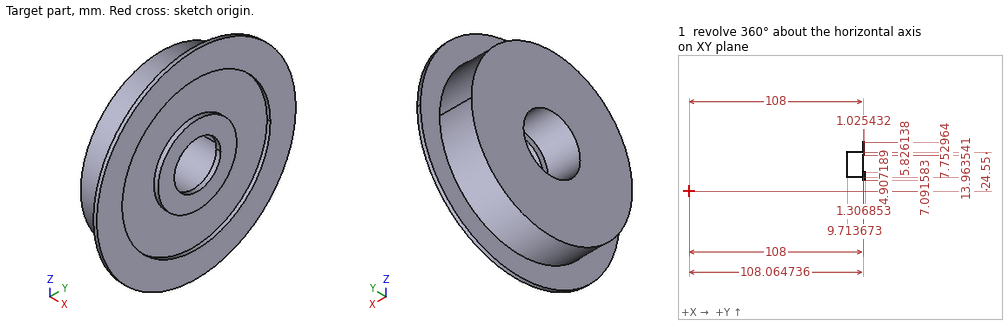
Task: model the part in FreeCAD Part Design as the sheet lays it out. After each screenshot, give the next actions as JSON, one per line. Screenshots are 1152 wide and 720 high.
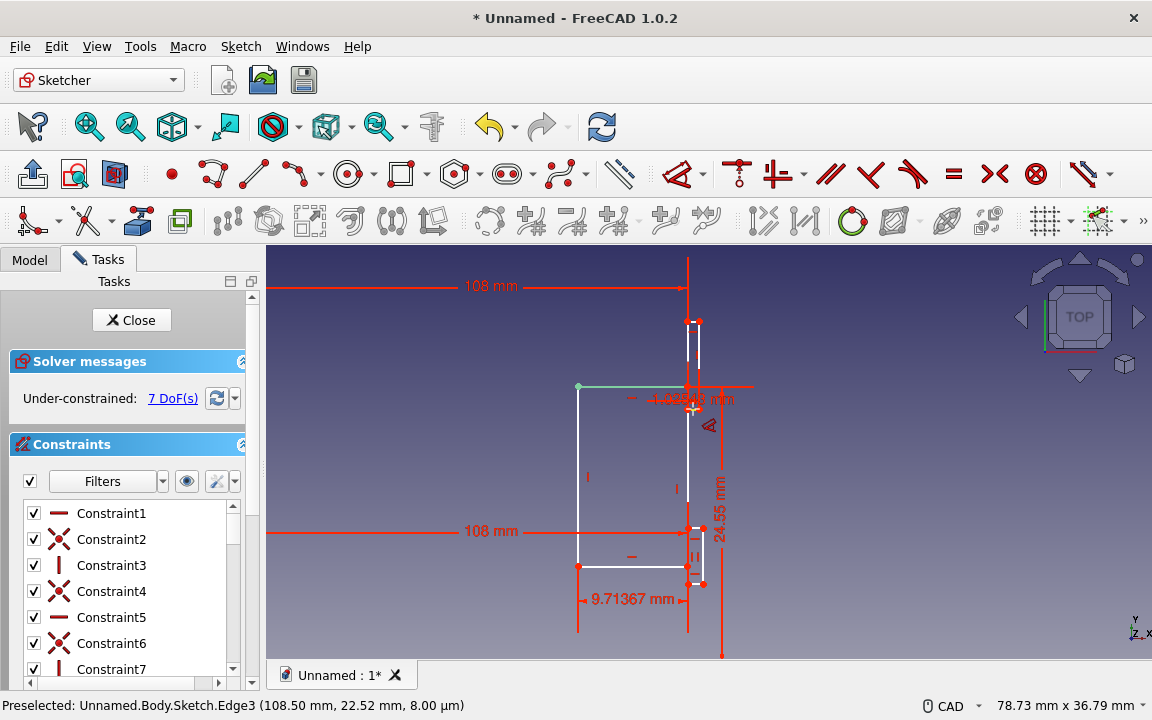
{"action": "left_click", "coordinate": [699, 383]}
{"action": "left_click", "coordinate": [733, 366]}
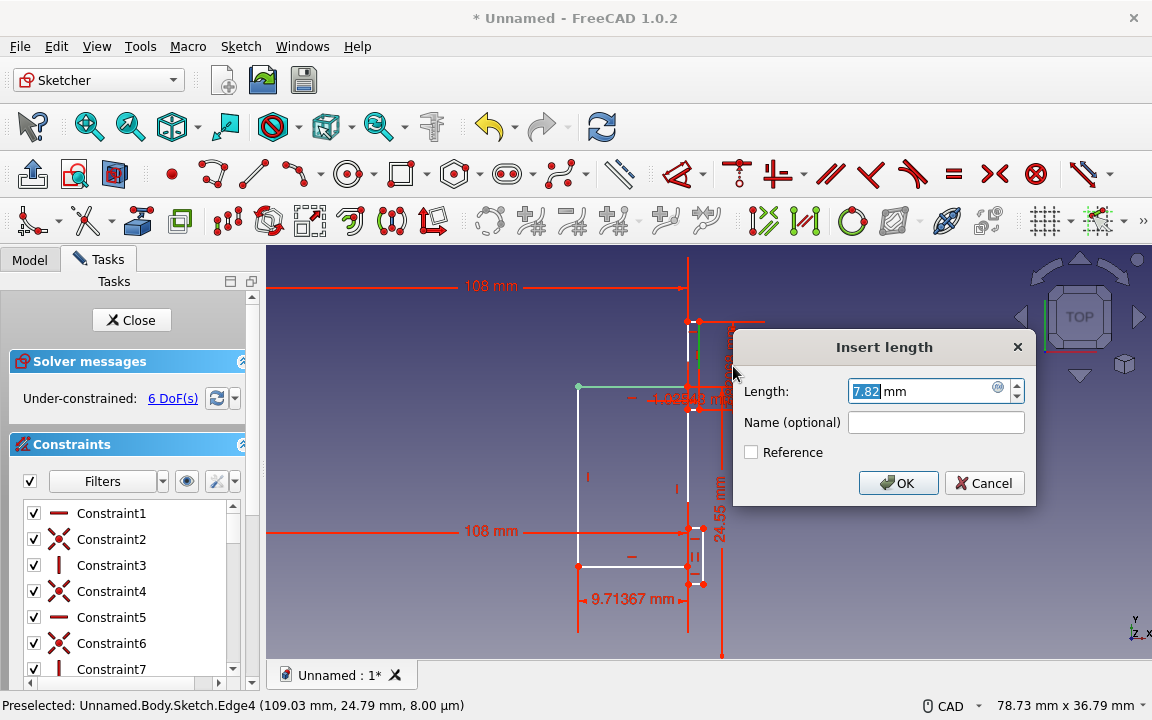
{"action": "type", "text": "7.752964"}
{"action": "key", "text": "Return"}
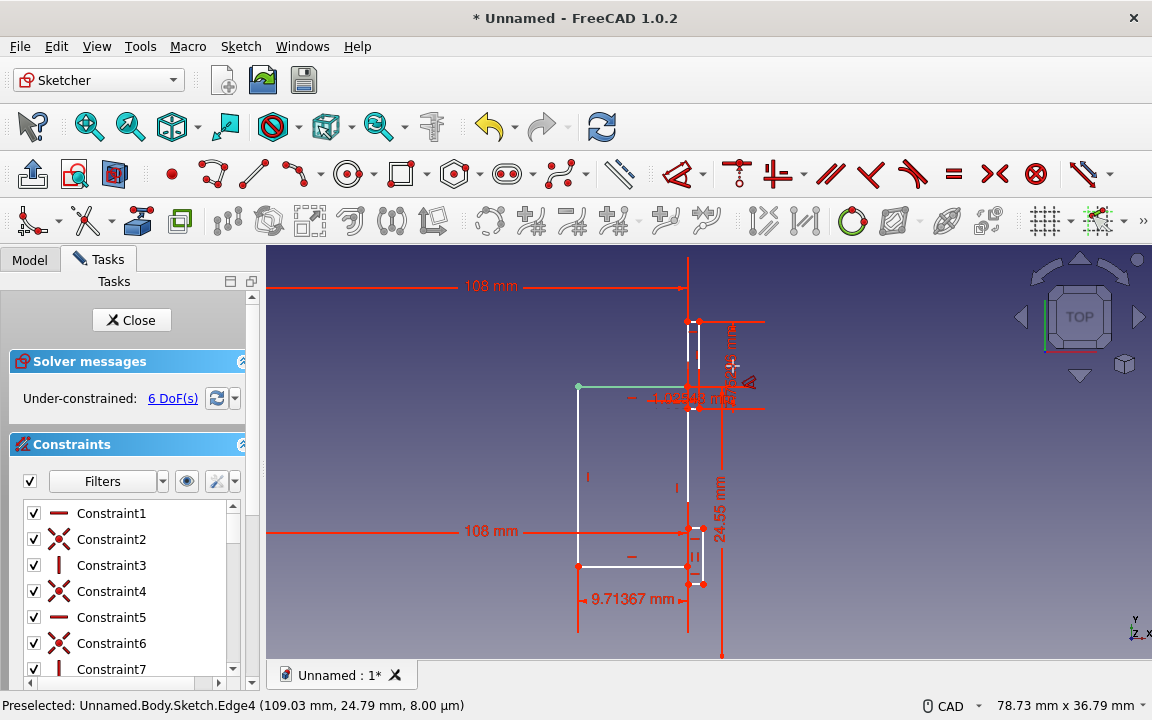
{"action": "left_click", "coordinate": [688, 341]}
{"action": "left_click", "coordinate": [722, 339]}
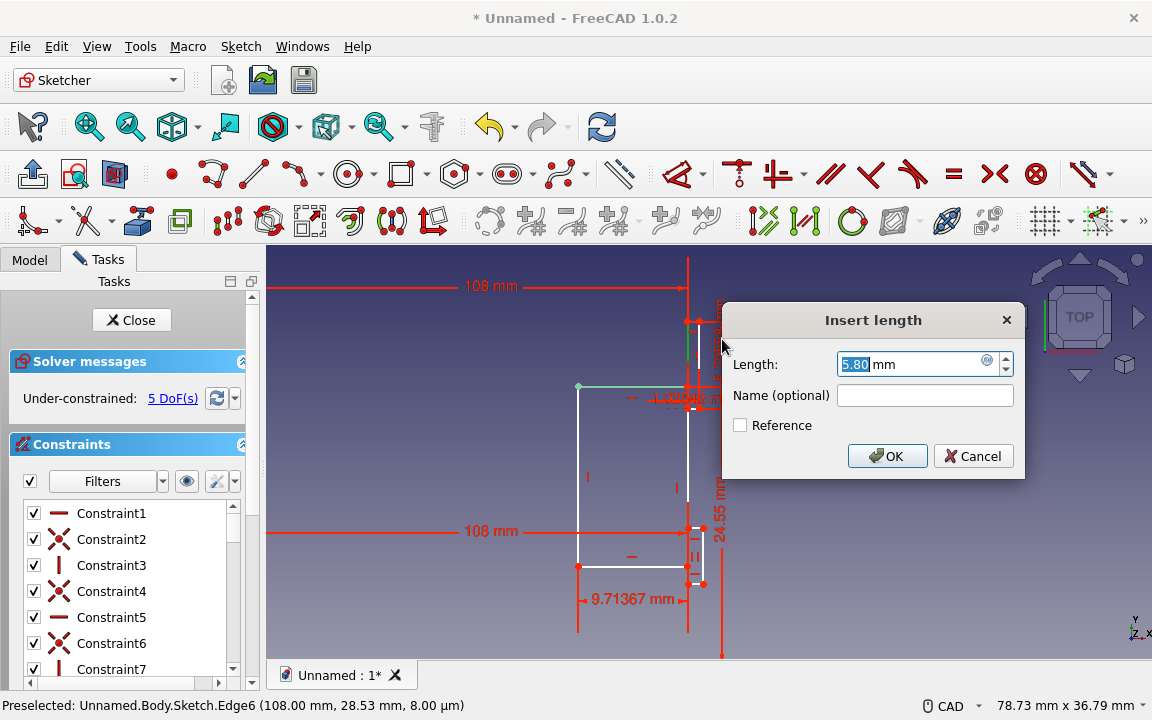
{"action": "type", "text": "5.826138"}
{"action": "key", "text": "Return"}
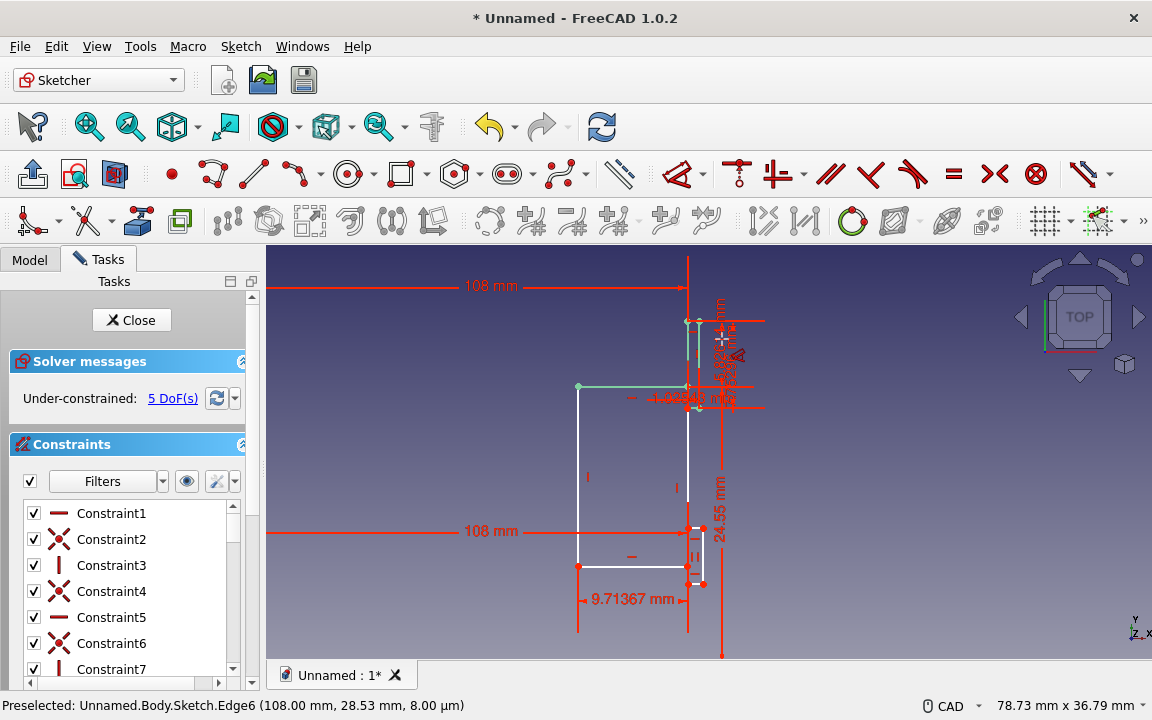
{"action": "scroll", "coordinate": [688, 573], "scroll_direction": "up", "scroll_amount": 4}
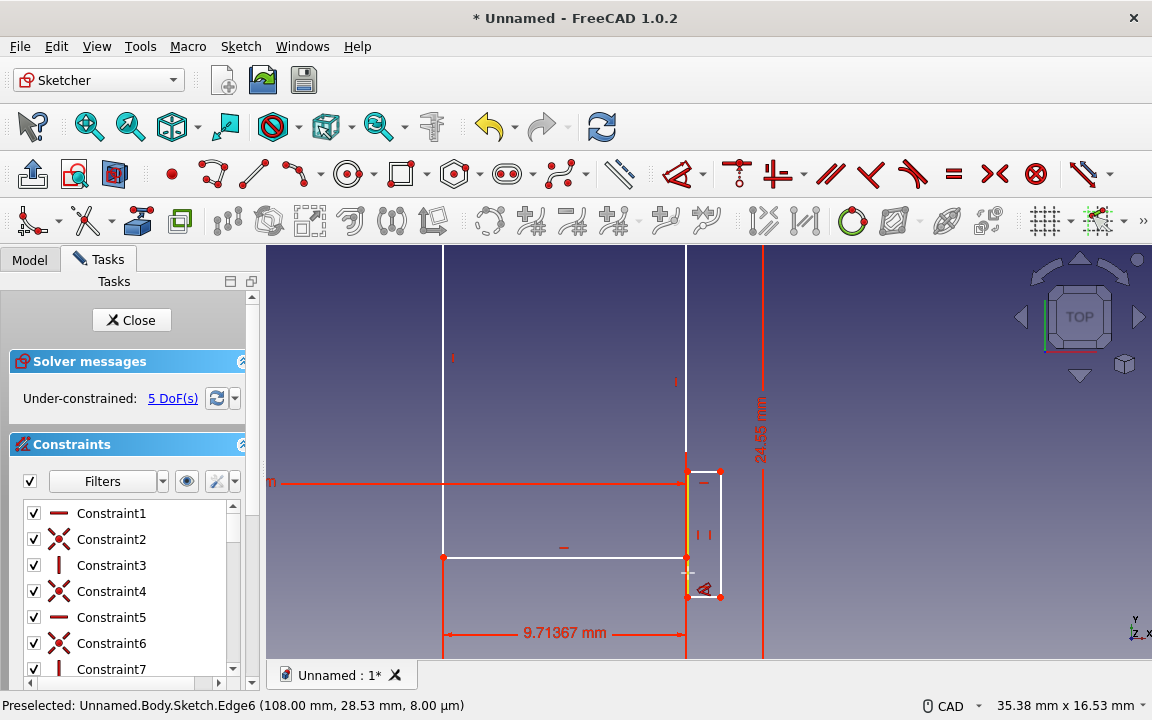
{"action": "left_click", "coordinate": [688, 572]}
{"action": "left_click", "coordinate": [654, 535]}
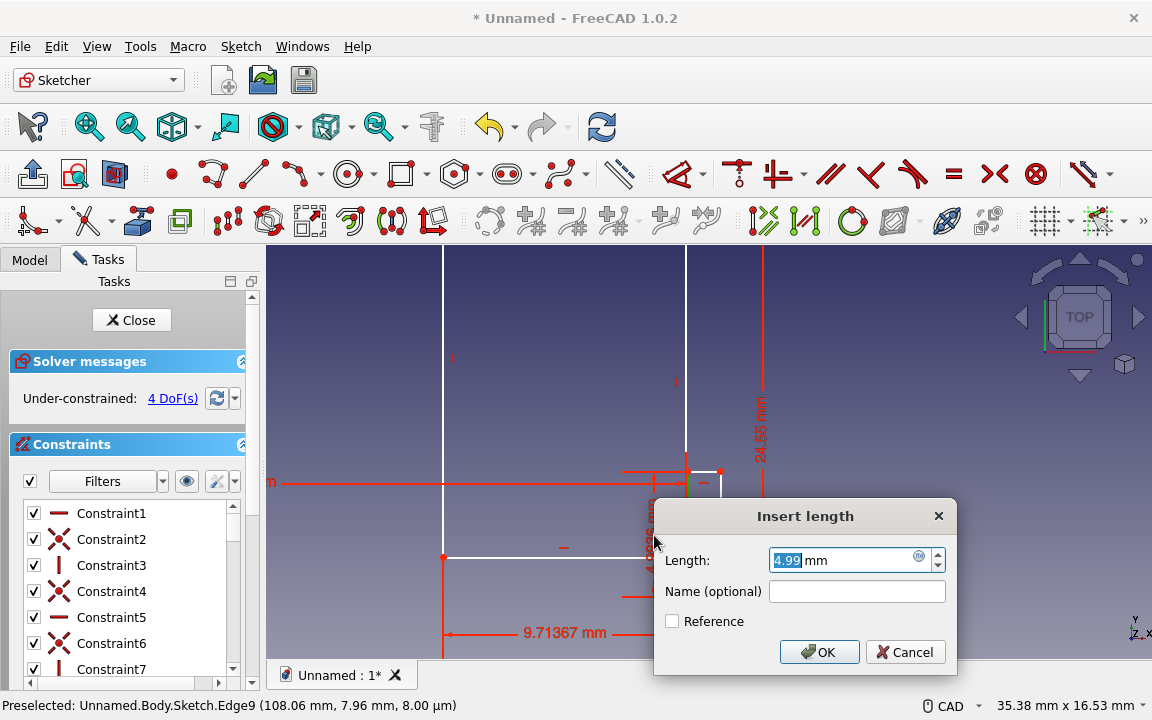
{"action": "type", "text": "4.907189"}
{"action": "key", "text": "Return"}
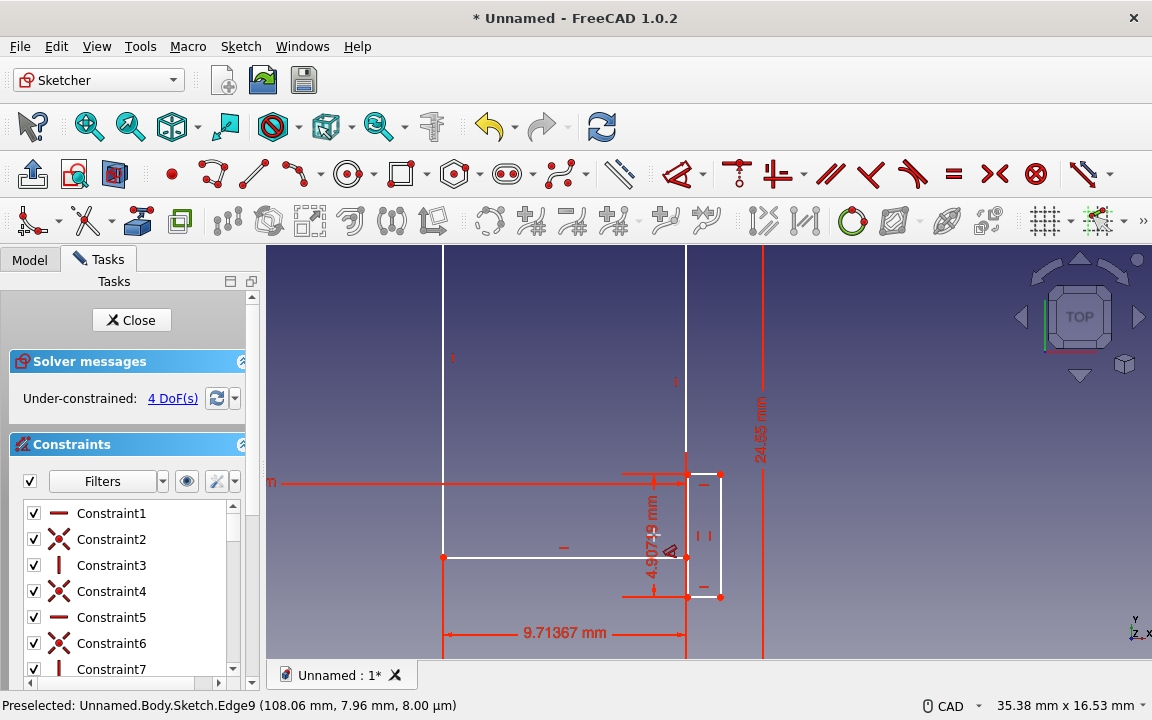
{"action": "scroll", "coordinate": [698, 597], "scroll_direction": "up", "scroll_amount": 2}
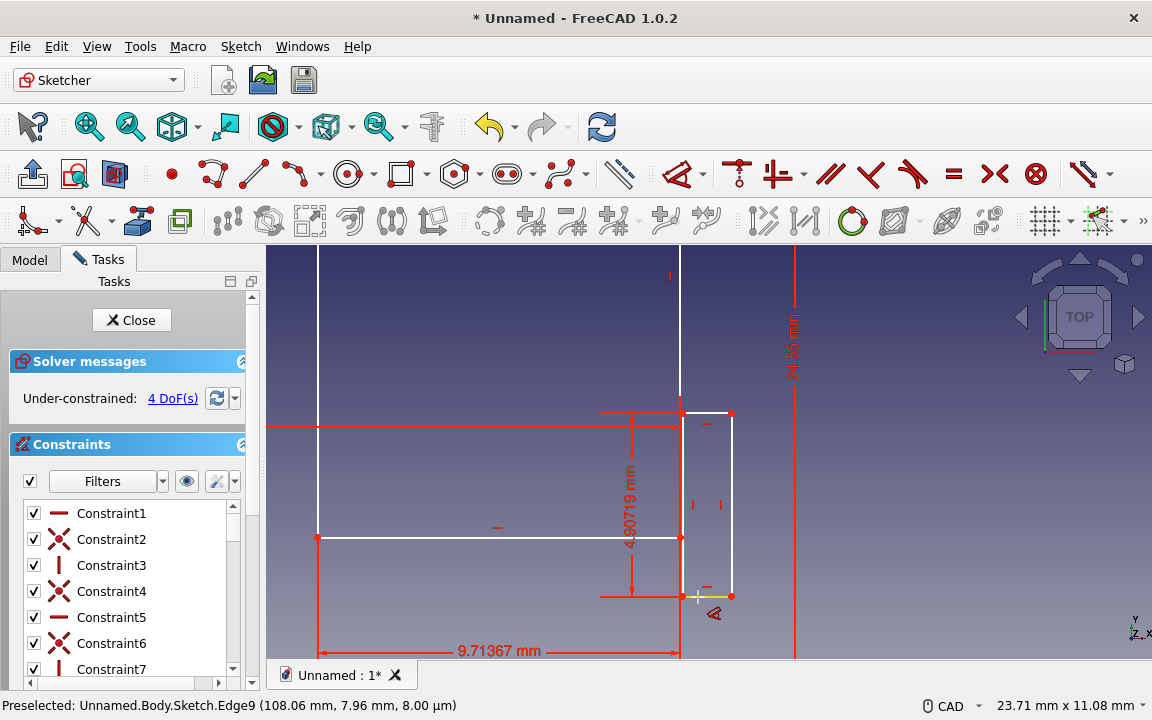
{"action": "left_click", "coordinate": [697, 597]}
{"action": "left_click", "coordinate": [707, 631]}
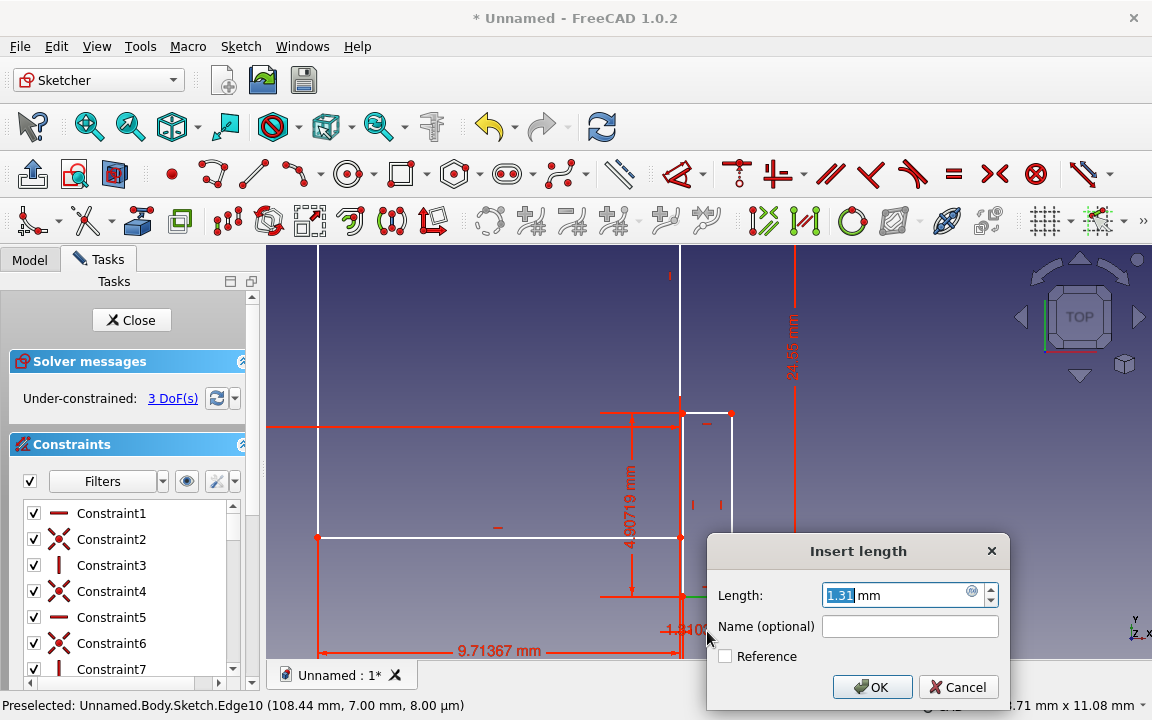
{"action": "type", "text": "1.306853"}
{"action": "key", "text": "Return"}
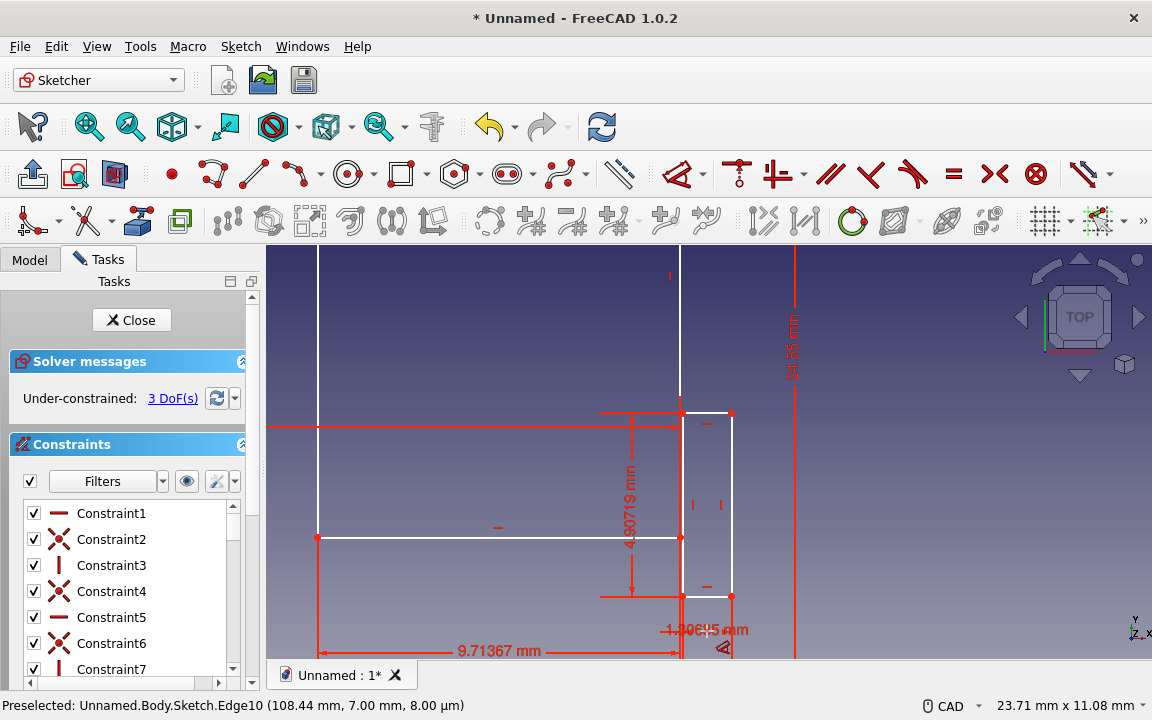
{"action": "left_click", "coordinate": [680, 380]}
{"action": "left_click", "coordinate": [714, 345]}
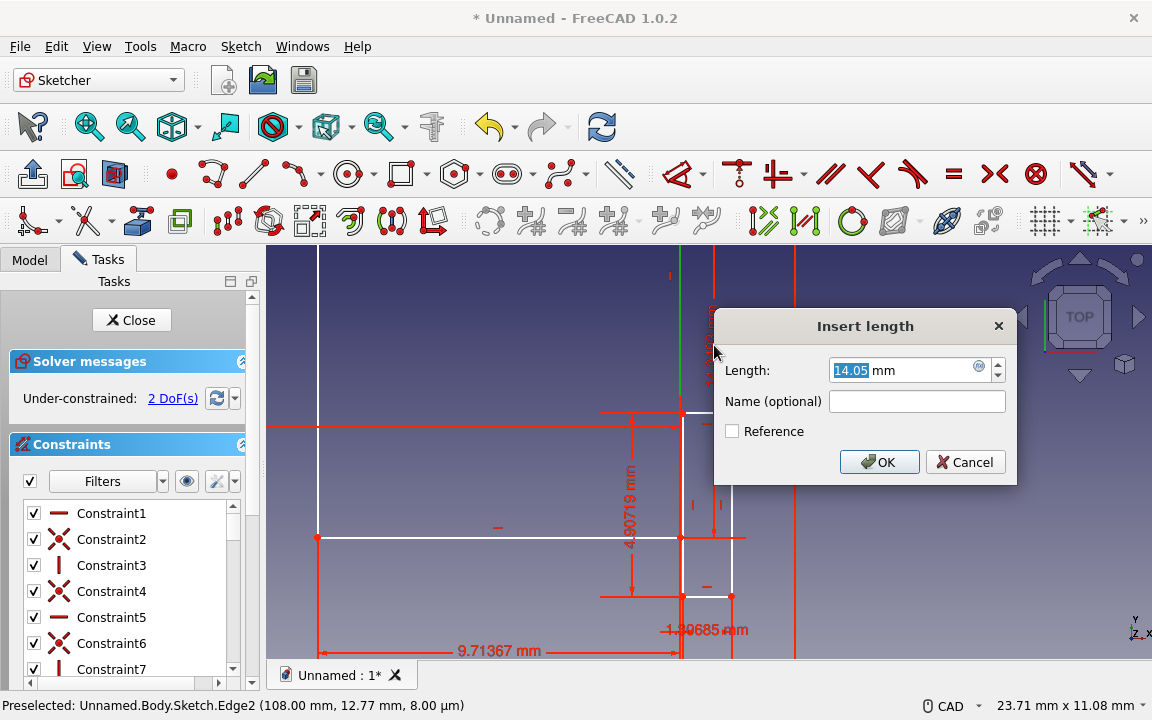
{"action": "type", "text": "13.963541"}
{"action": "key", "text": "Return"}